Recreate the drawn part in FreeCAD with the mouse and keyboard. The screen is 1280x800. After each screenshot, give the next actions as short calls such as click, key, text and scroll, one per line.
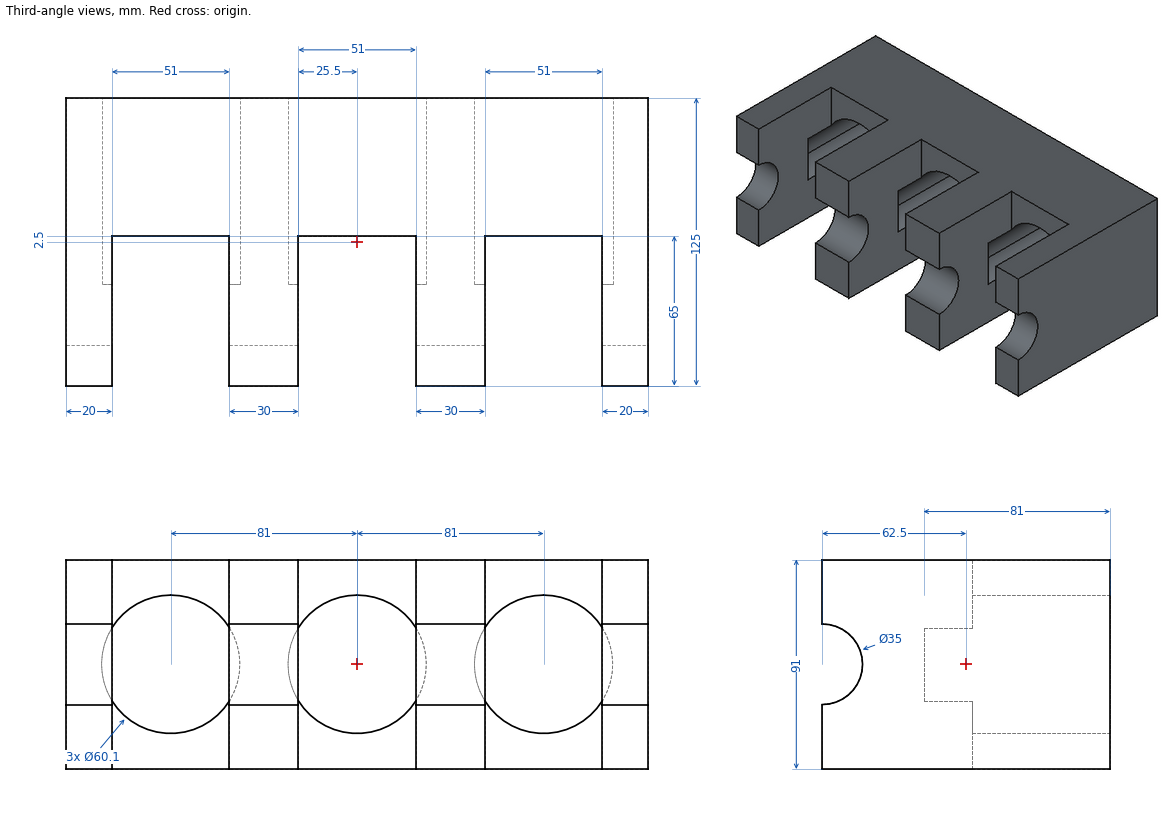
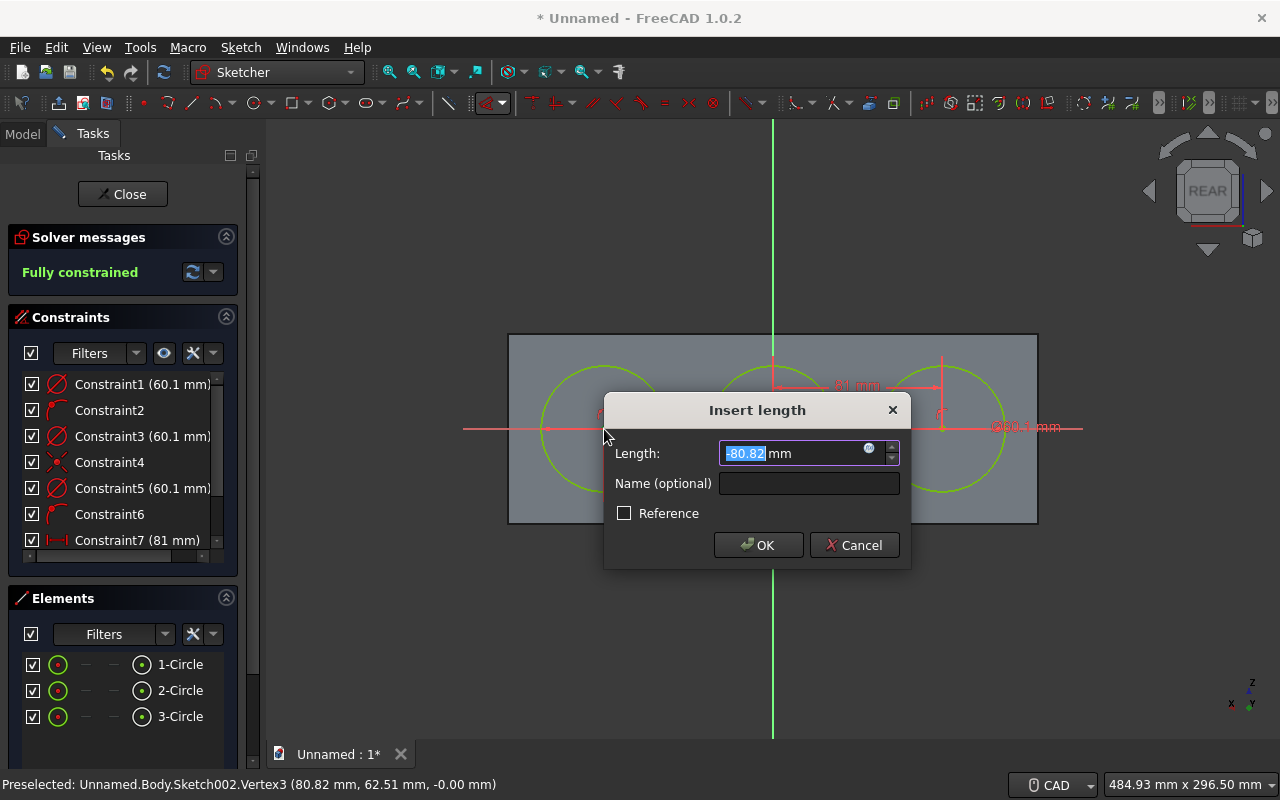
text(-81)
key(Return)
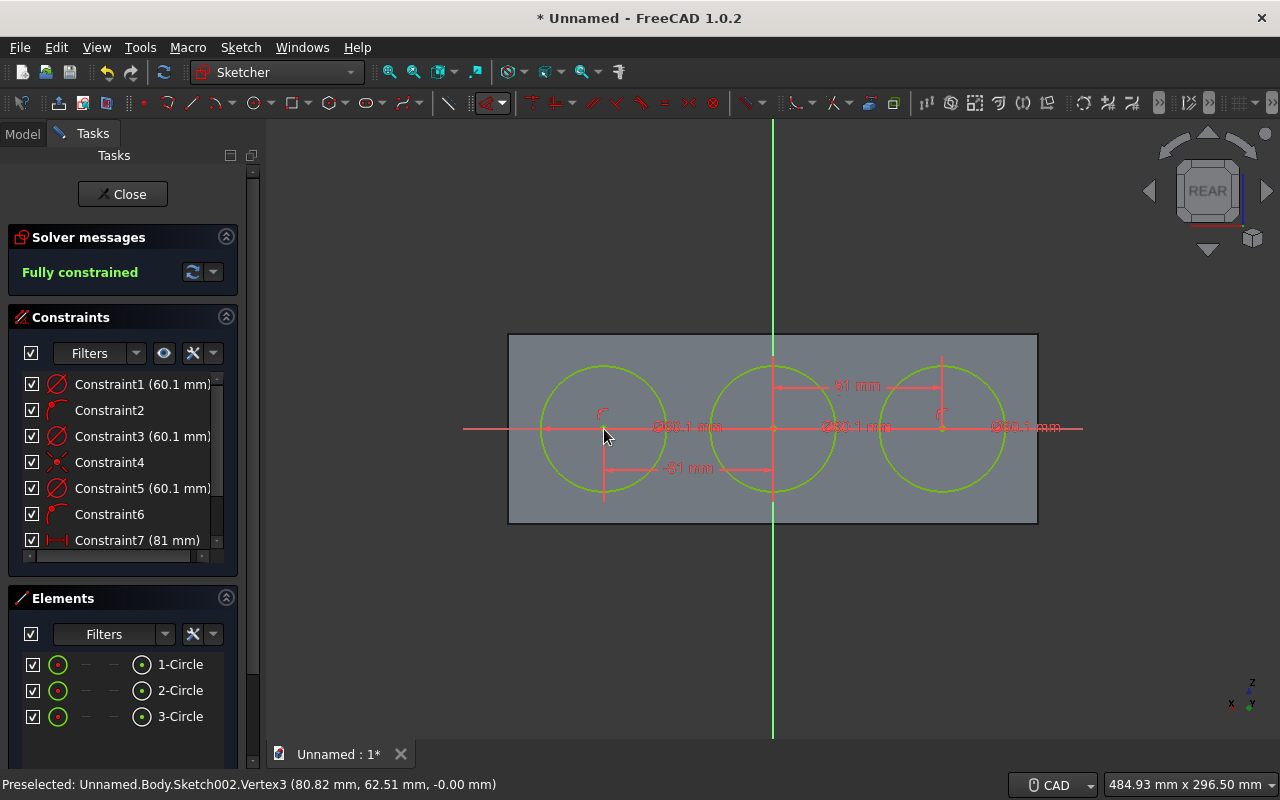
click(123, 194)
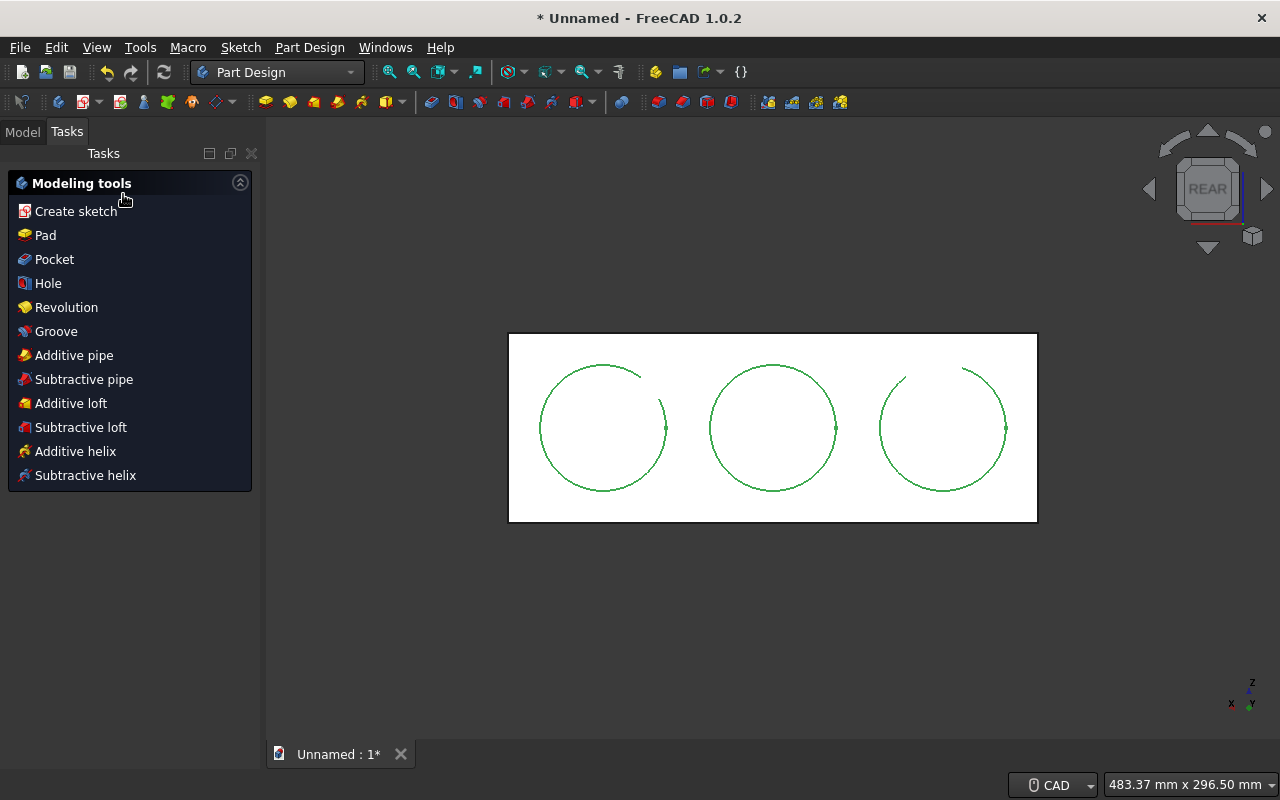
click(432, 102)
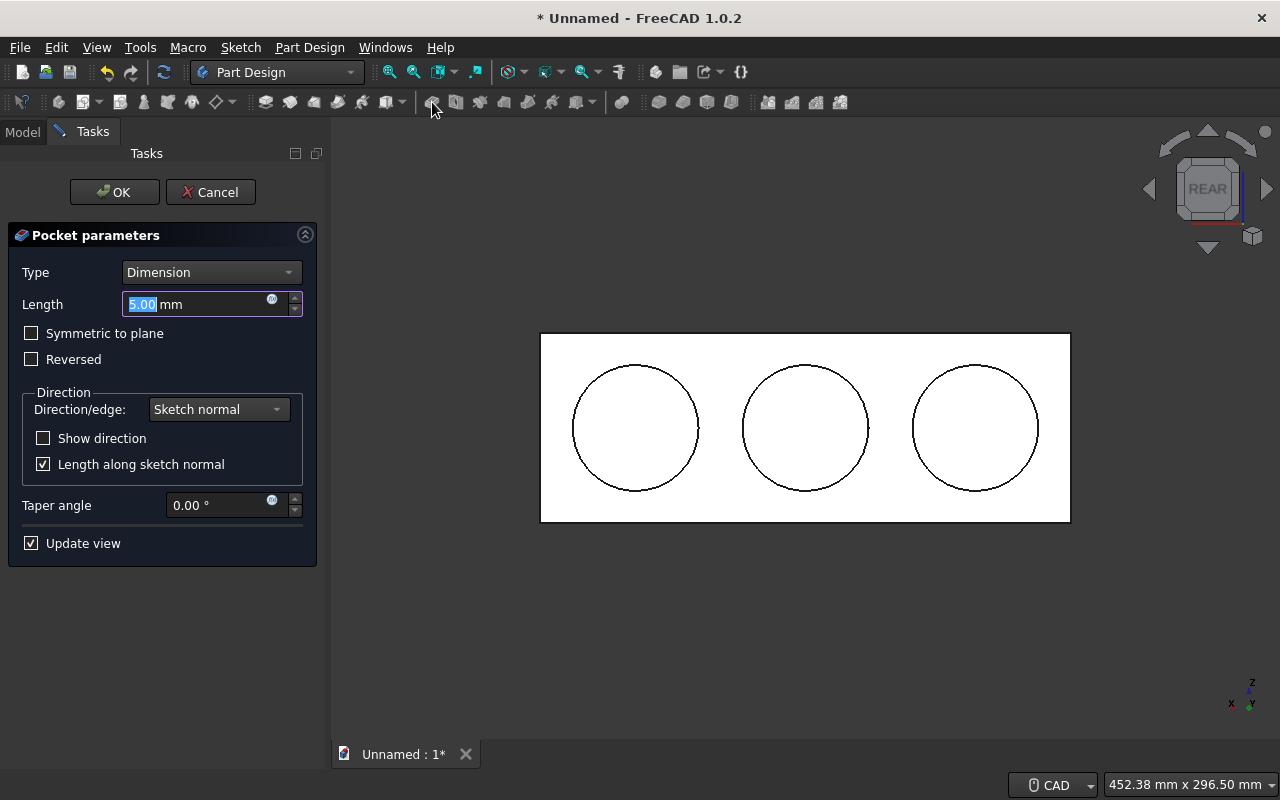
text(81)
key(Tab)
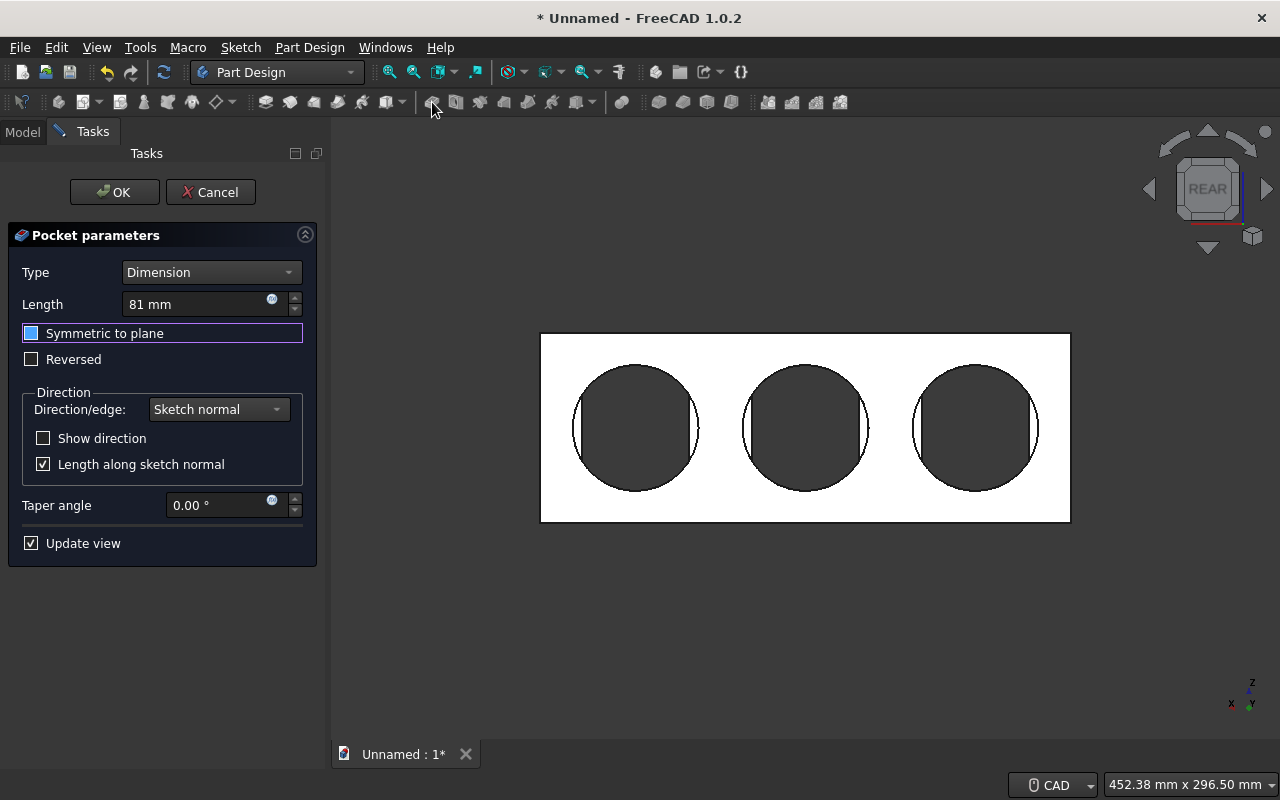
click(115, 192)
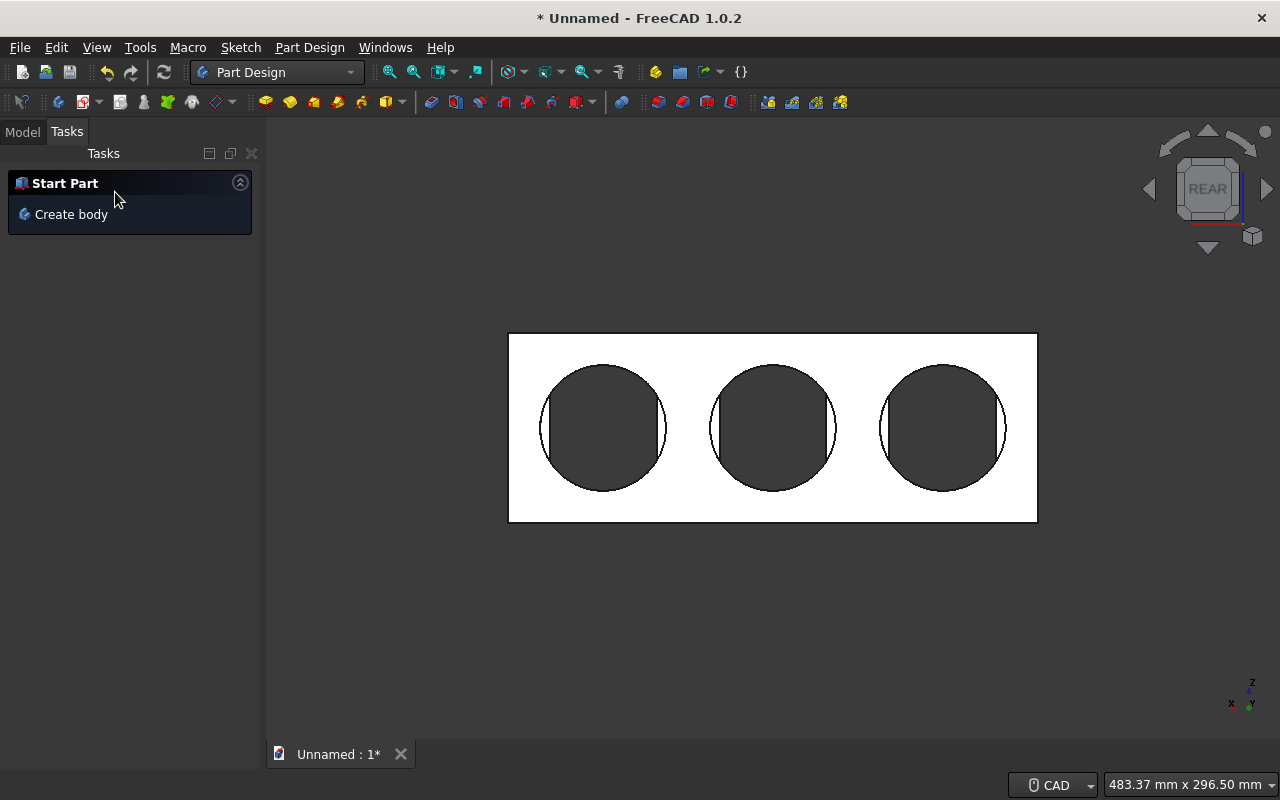
key(0)